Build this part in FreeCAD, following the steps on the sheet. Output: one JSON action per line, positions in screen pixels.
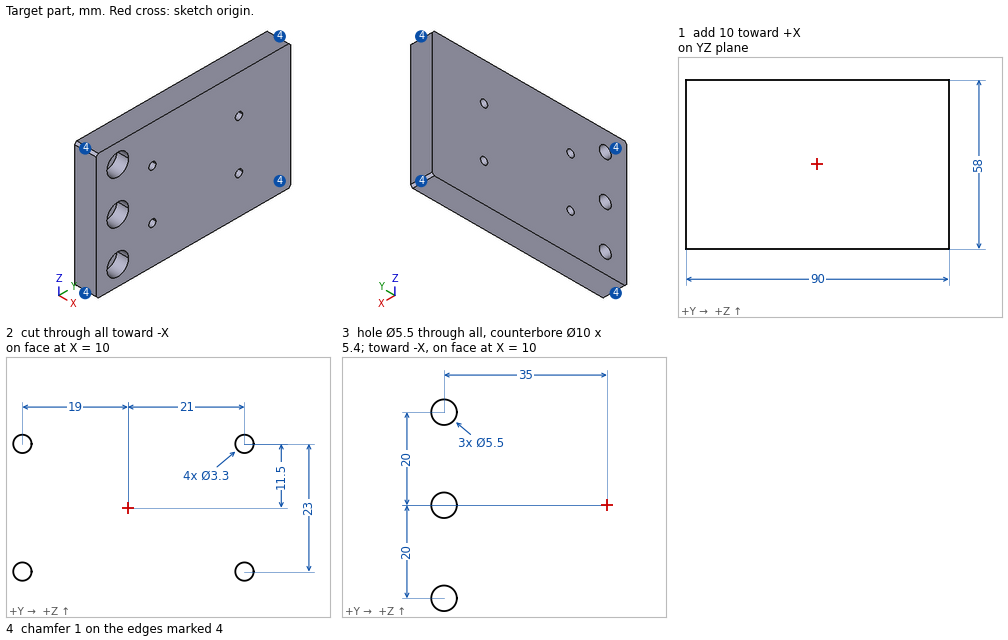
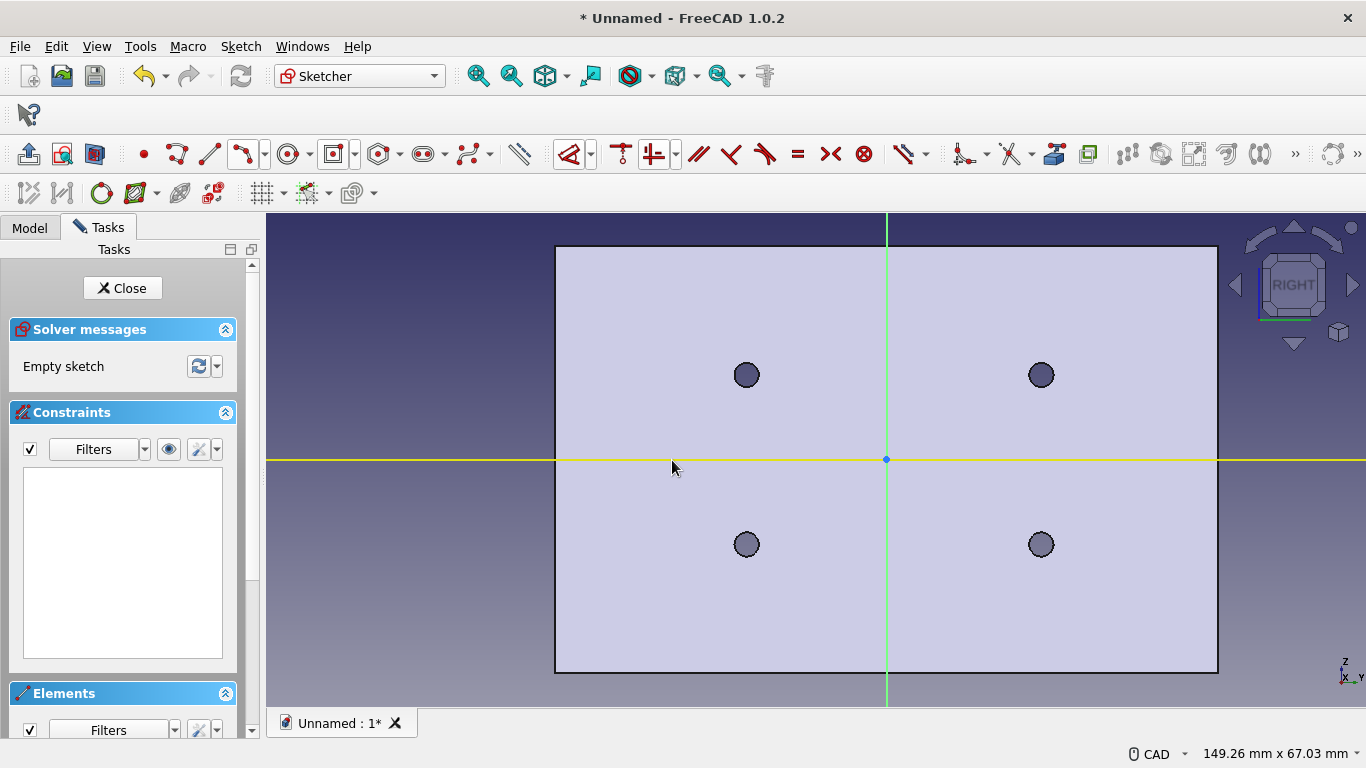
{"action": "left_click", "coordinate": [288, 154]}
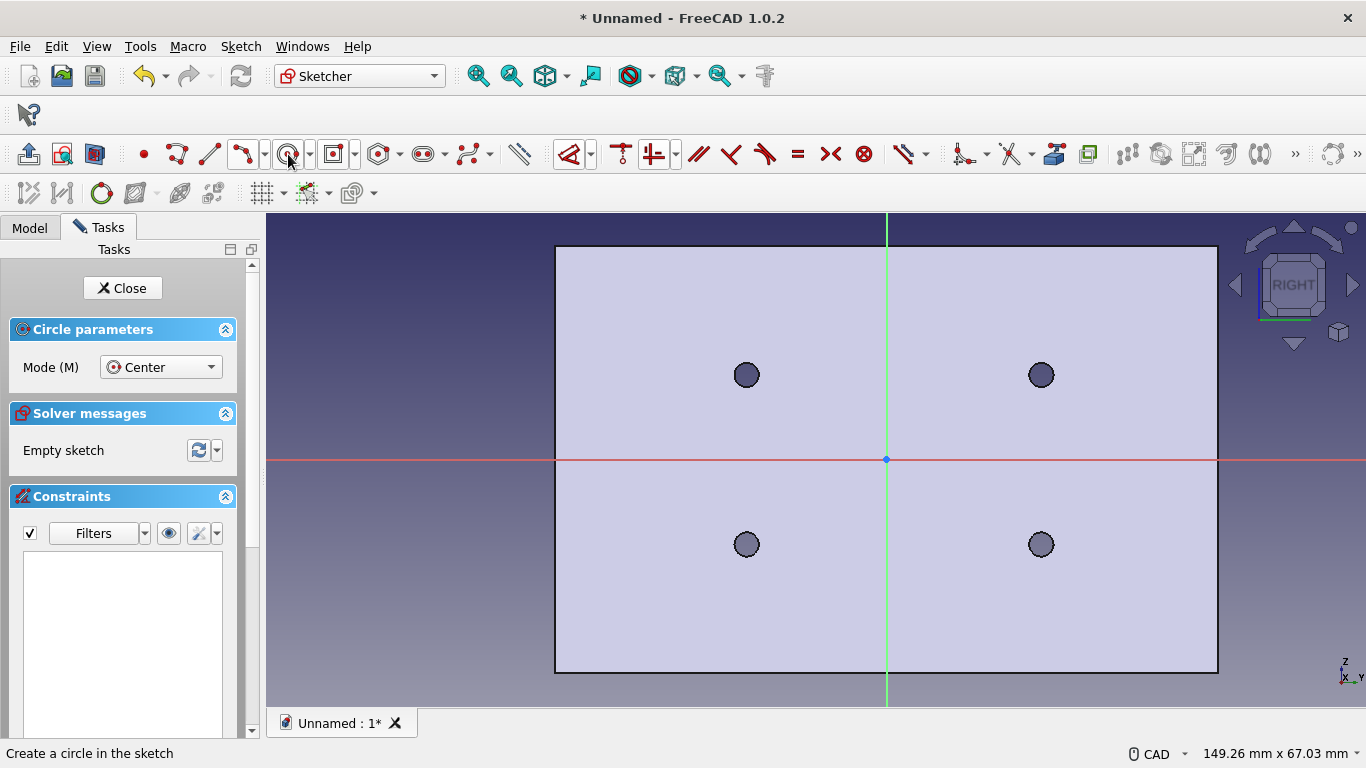
{"action": "left_click", "coordinate": [629, 312]}
{"action": "mouse_move", "coordinate": [643, 298]}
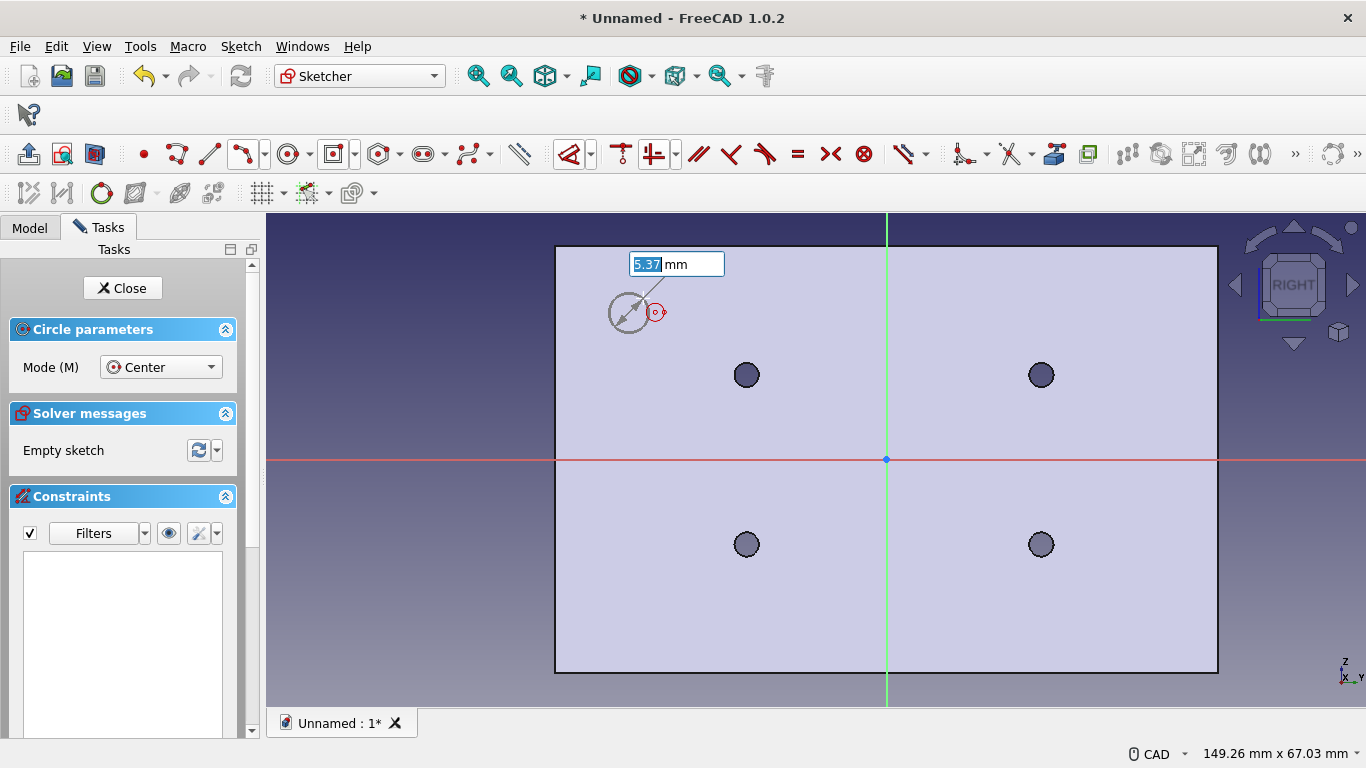
{"action": "type", "text": "5.5"}
{"action": "key", "text": "Return"}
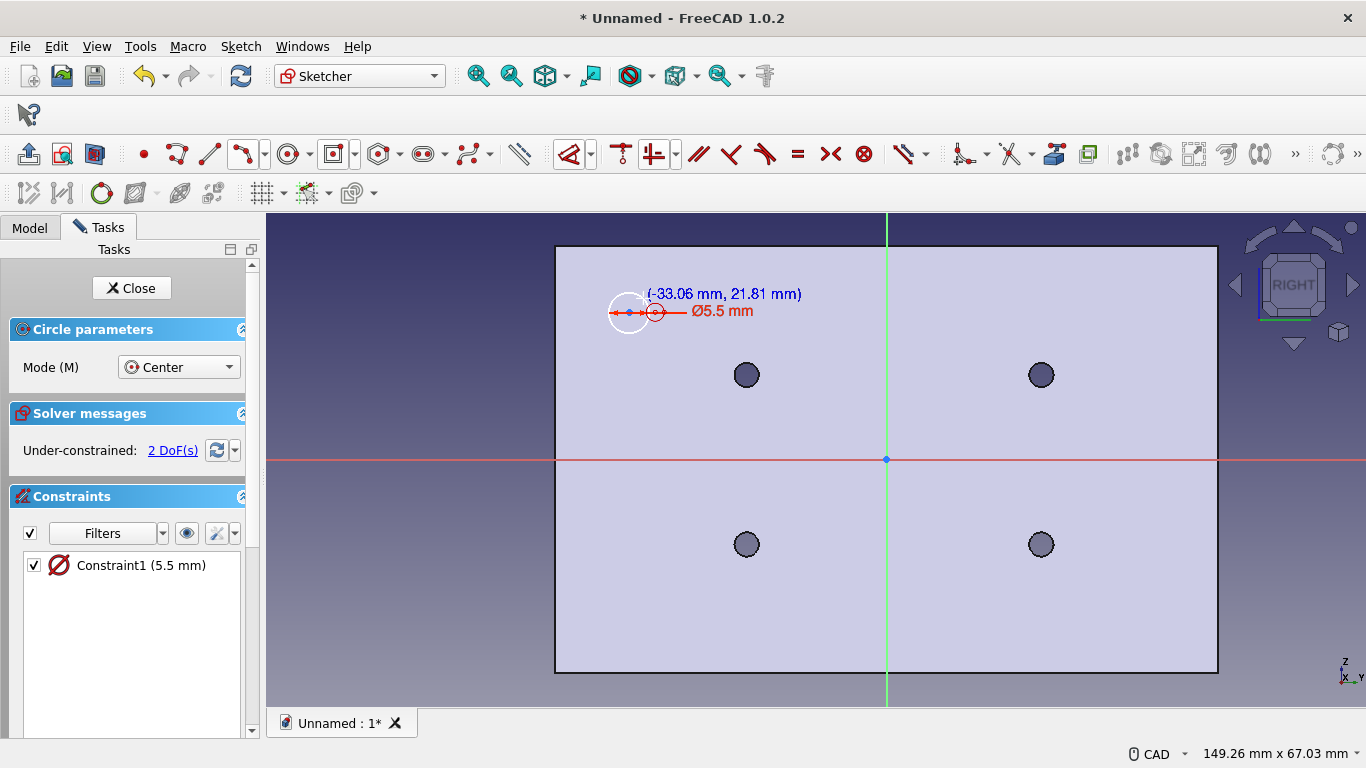
{"action": "left_click", "coordinate": [629, 460]}
{"action": "mouse_move", "coordinate": [643, 445]}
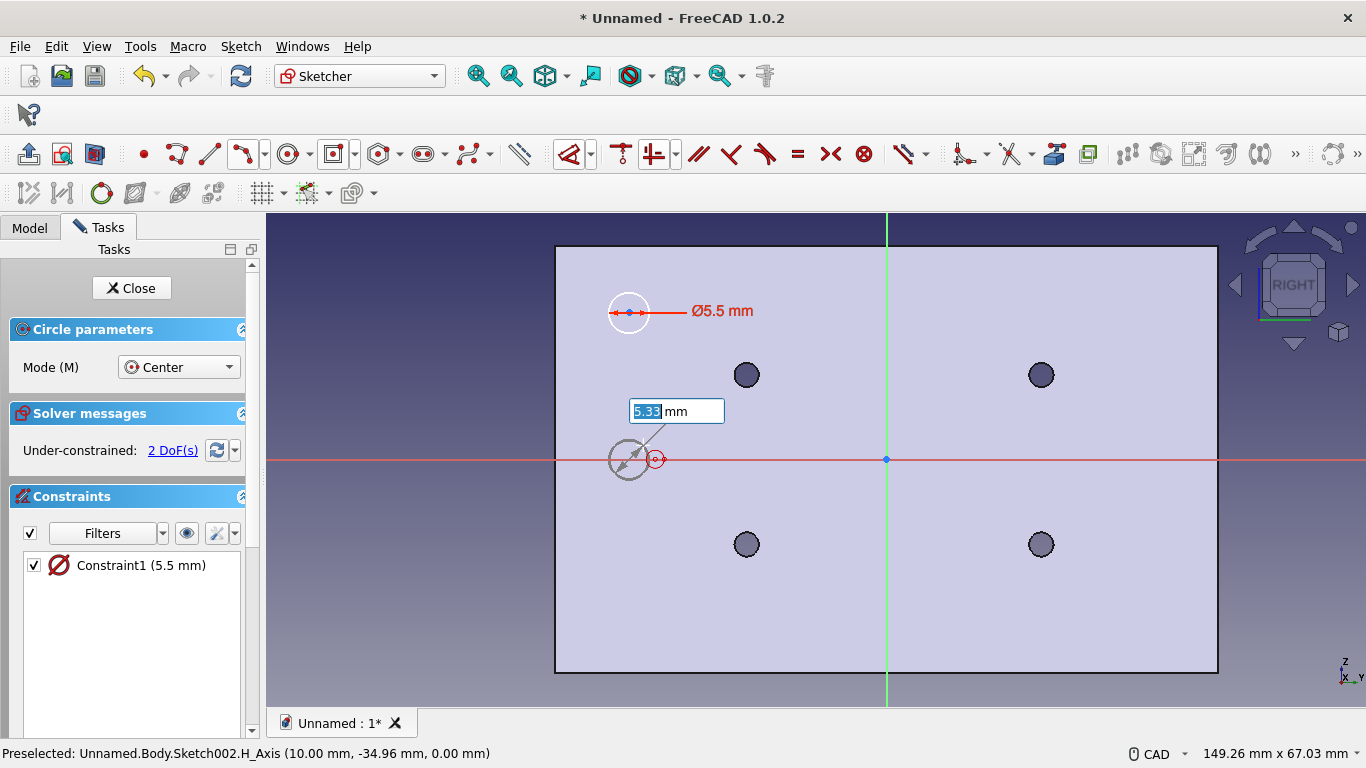
{"action": "type", "text": "5.5"}
{"action": "key", "text": "Return"}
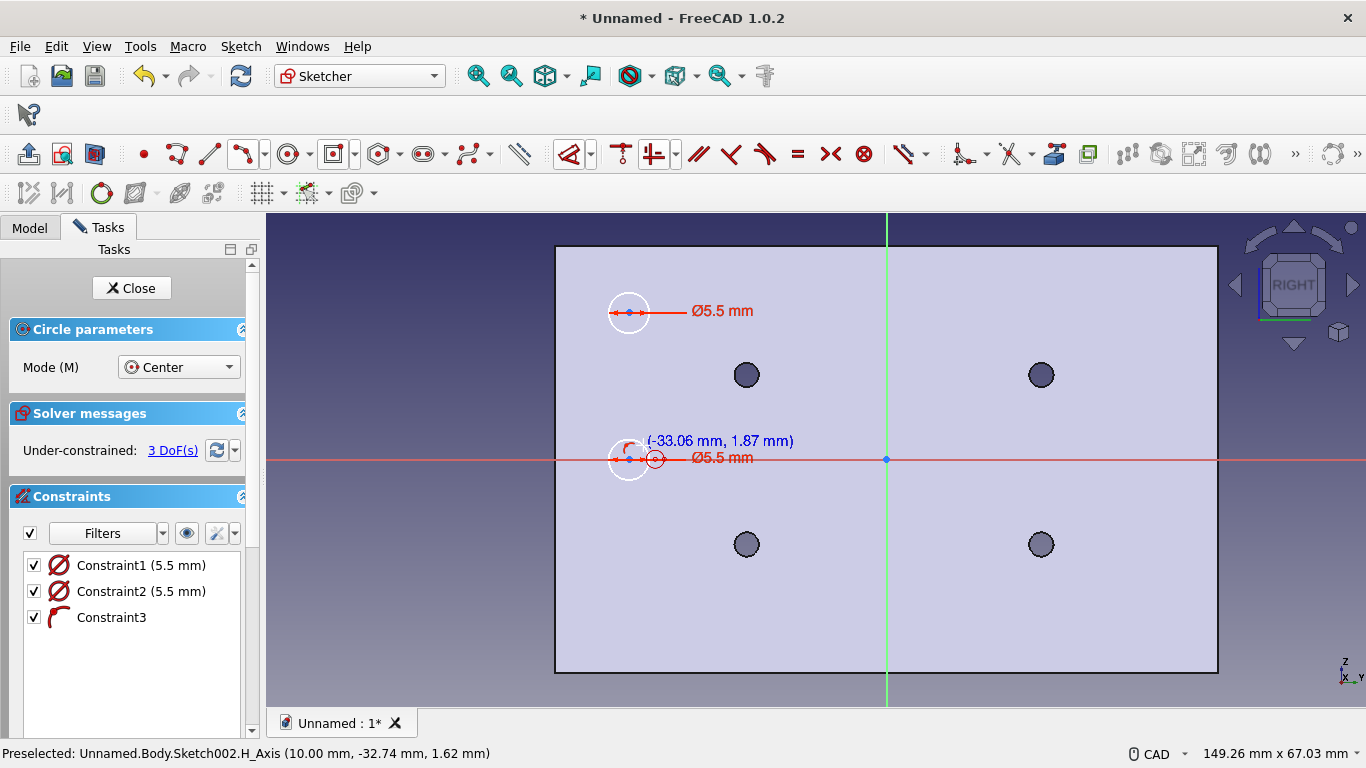
{"action": "left_click", "coordinate": [629, 607]}
{"action": "mouse_move", "coordinate": [643, 593]}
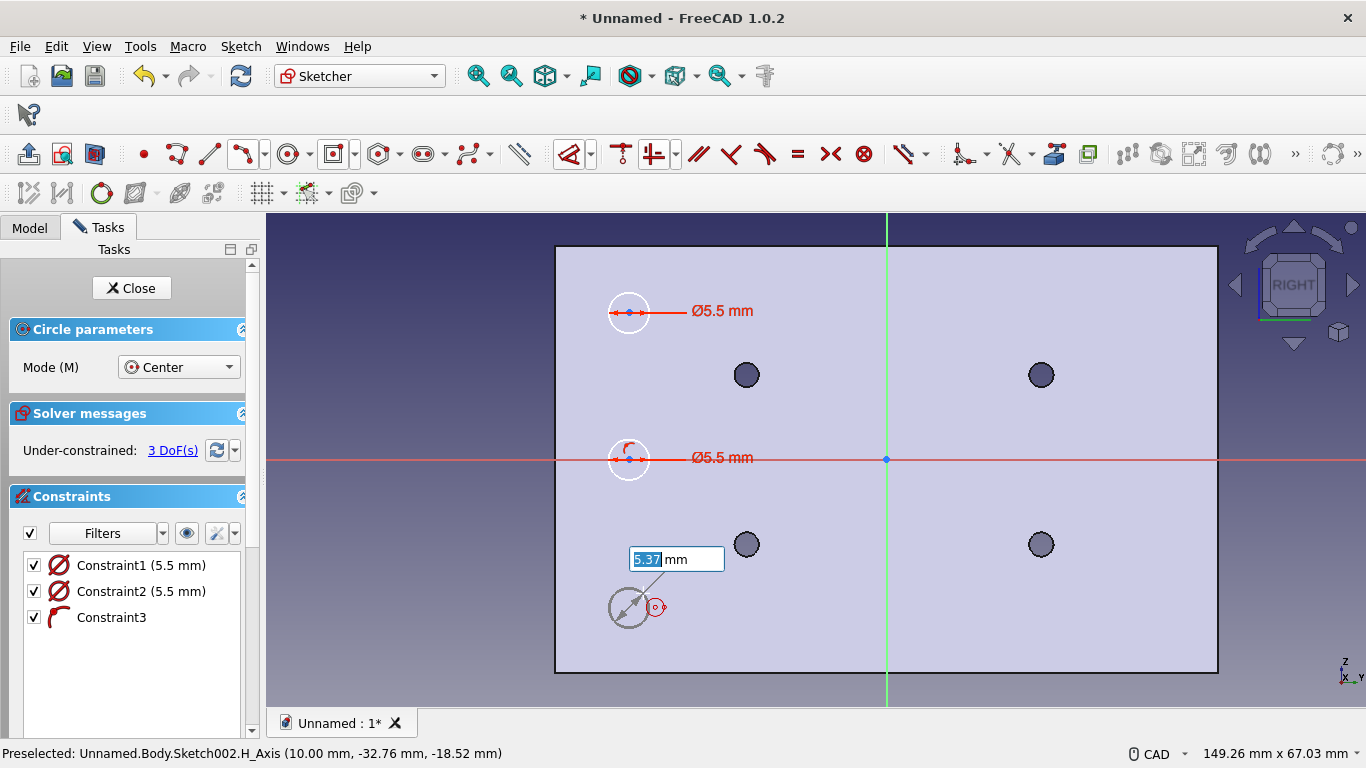
{"action": "type", "text": "5.5"}
{"action": "key", "text": "Return"}
{"action": "key", "text": "Escape"}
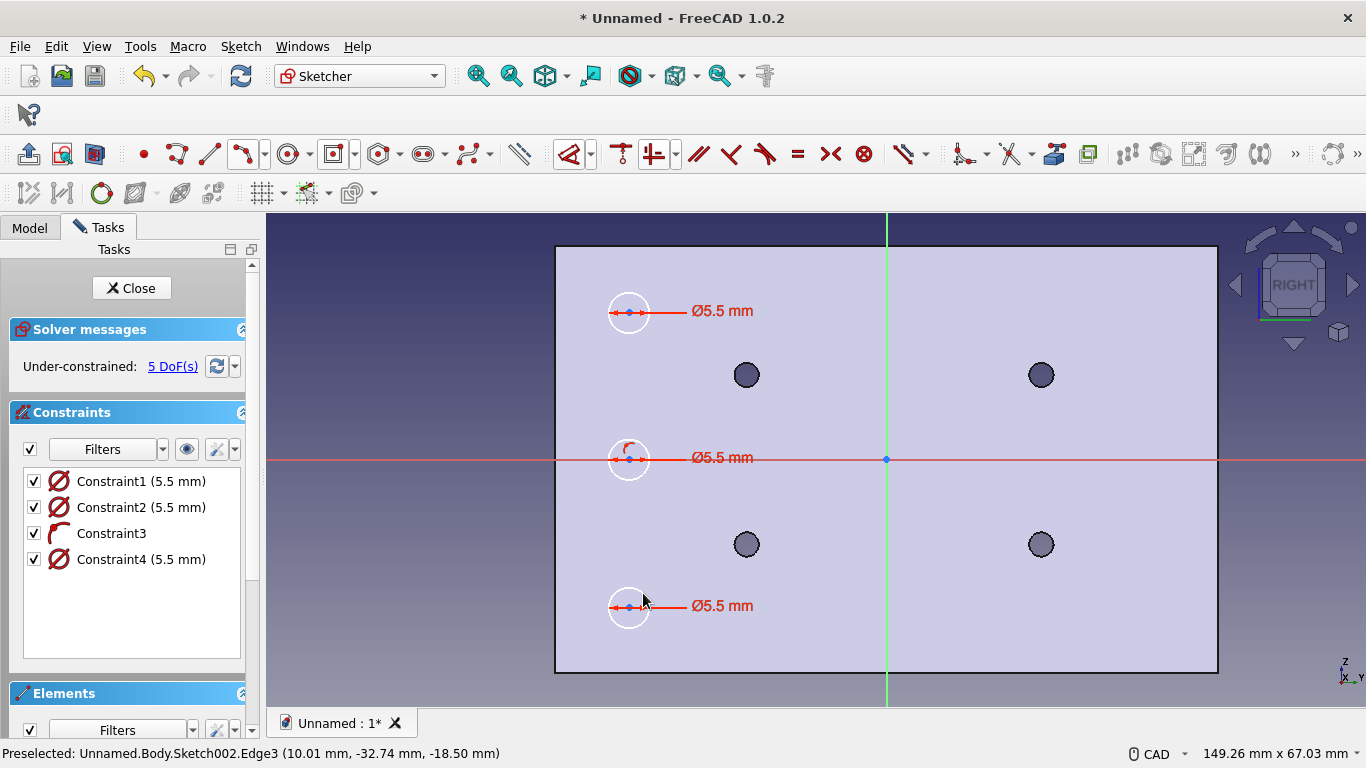
{"action": "left_click", "coordinate": [629, 313]}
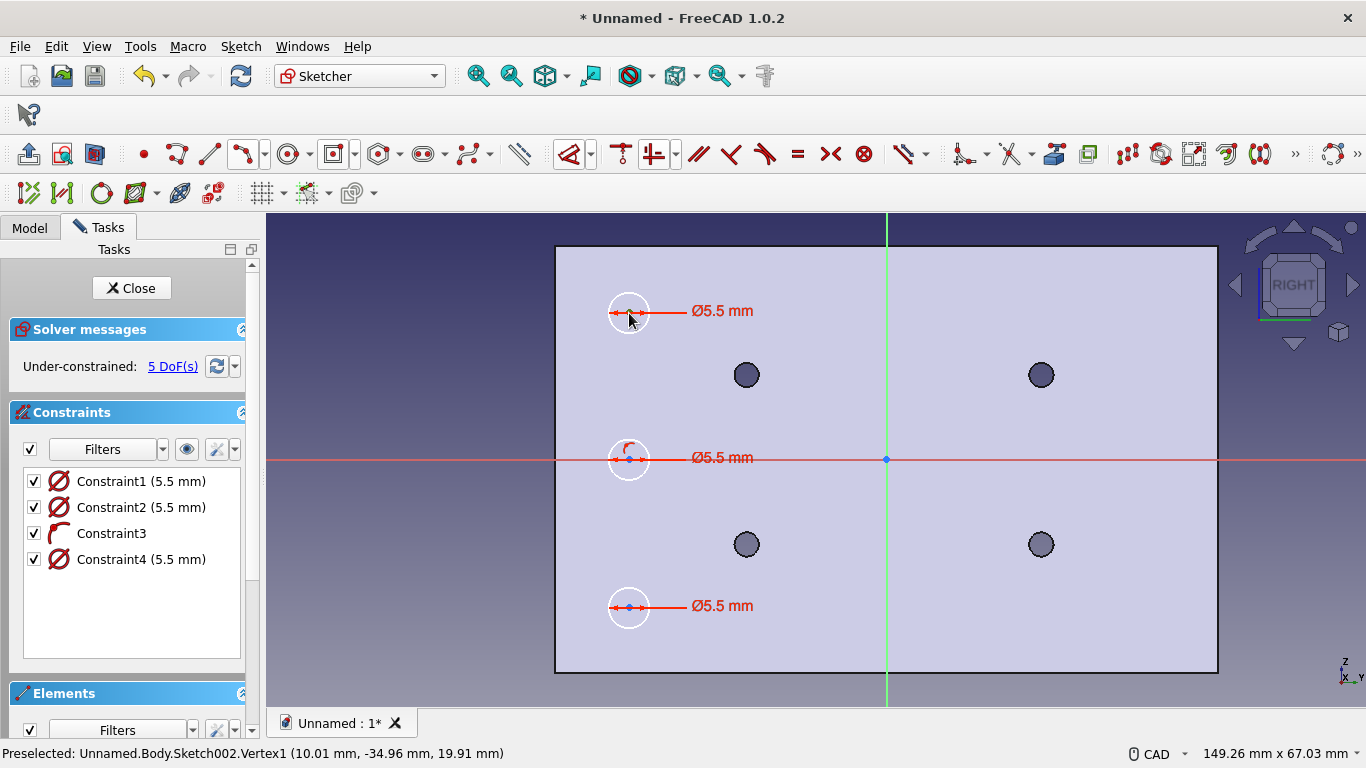
{"action": "left_click", "coordinate": [629, 460]}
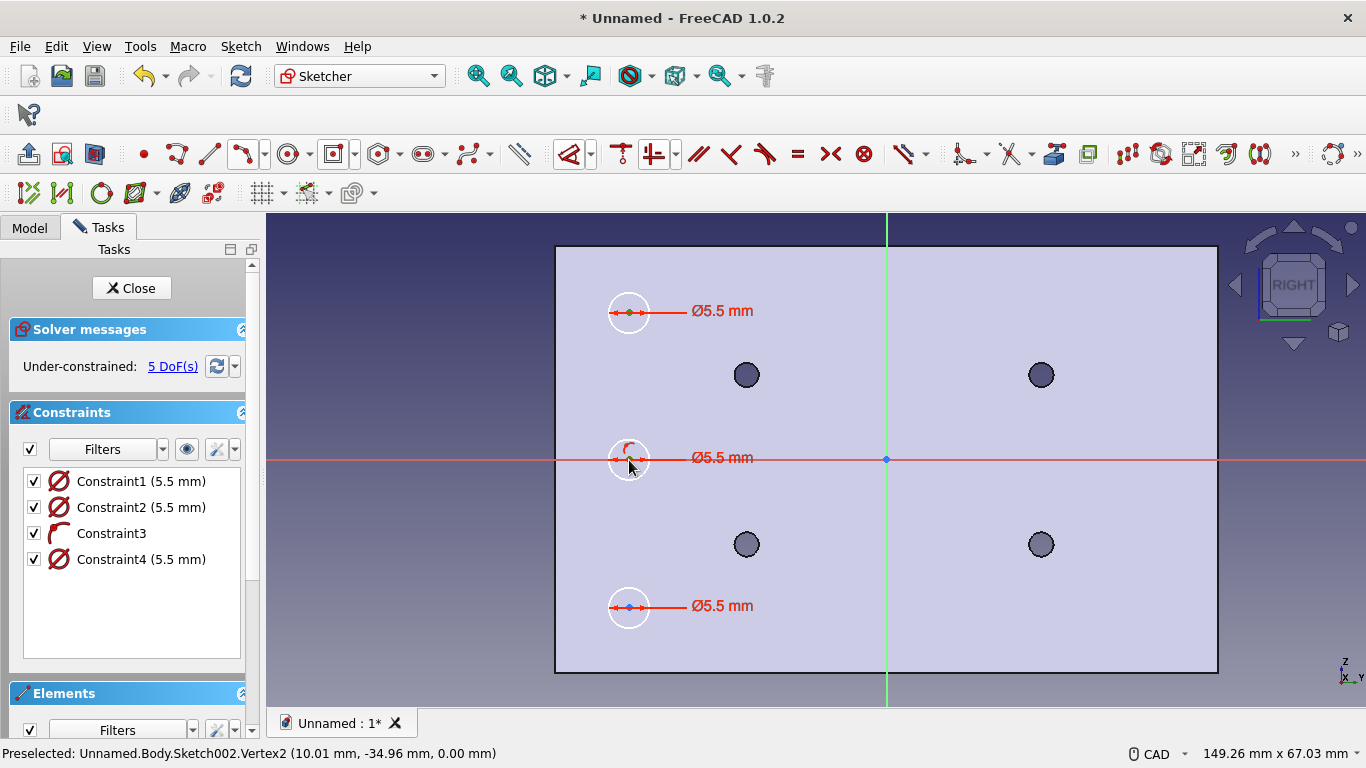
{"action": "left_click", "coordinate": [676, 154]}